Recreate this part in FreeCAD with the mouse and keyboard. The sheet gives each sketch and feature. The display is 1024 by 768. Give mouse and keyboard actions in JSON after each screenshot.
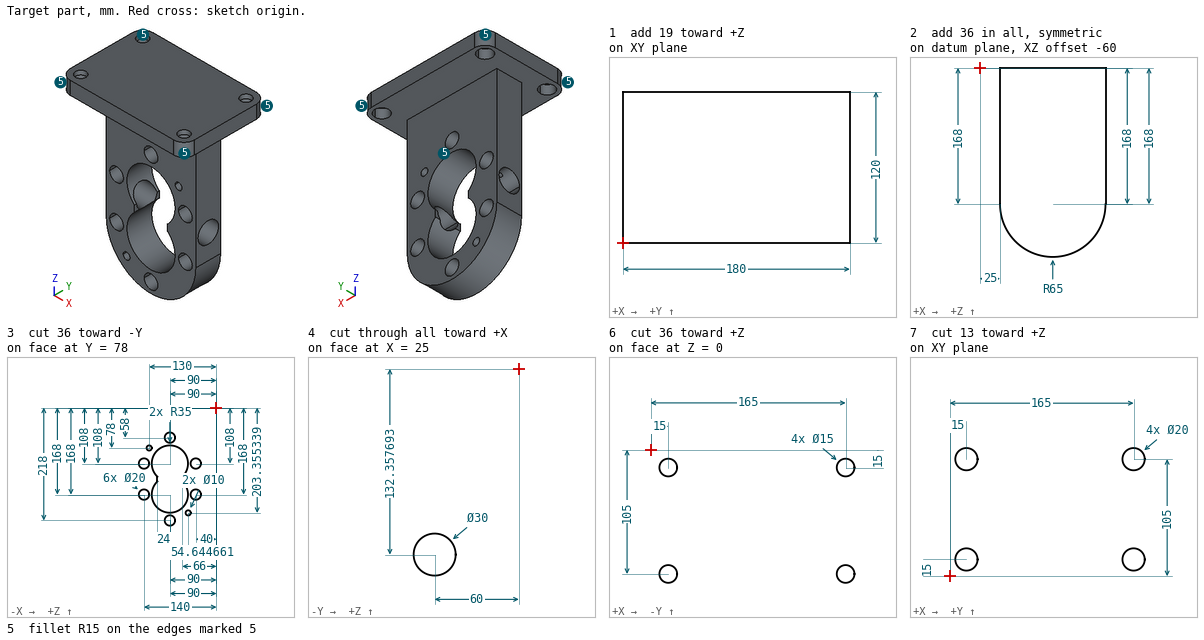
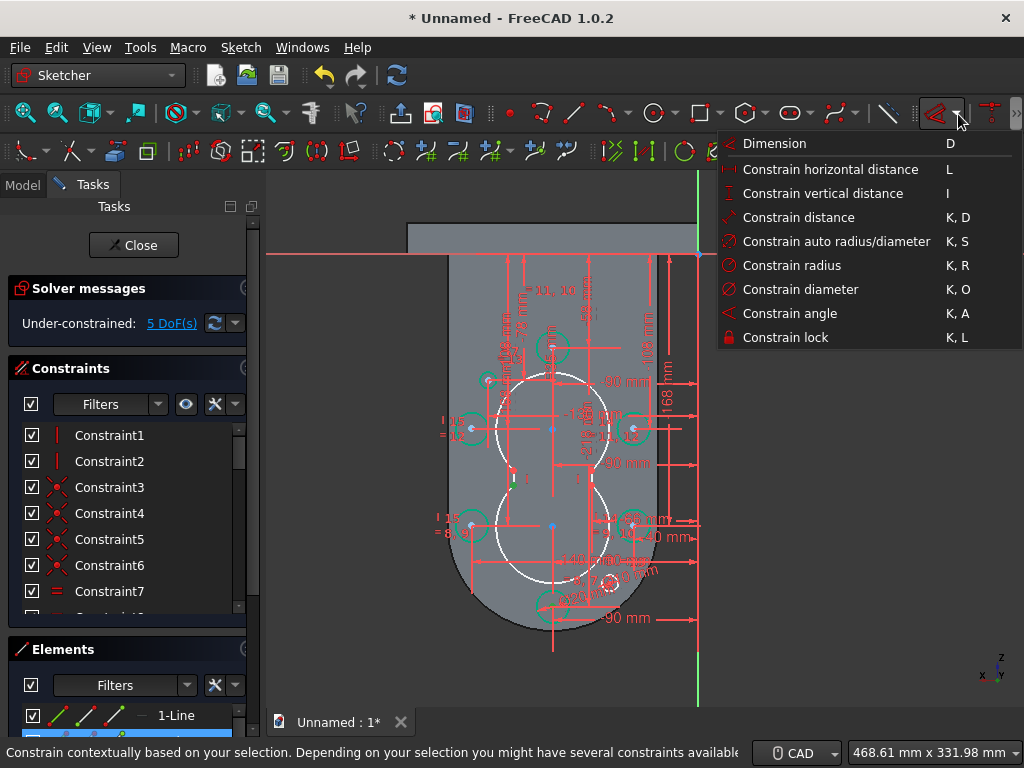
{"action": "left_click", "coordinate": [870, 169]}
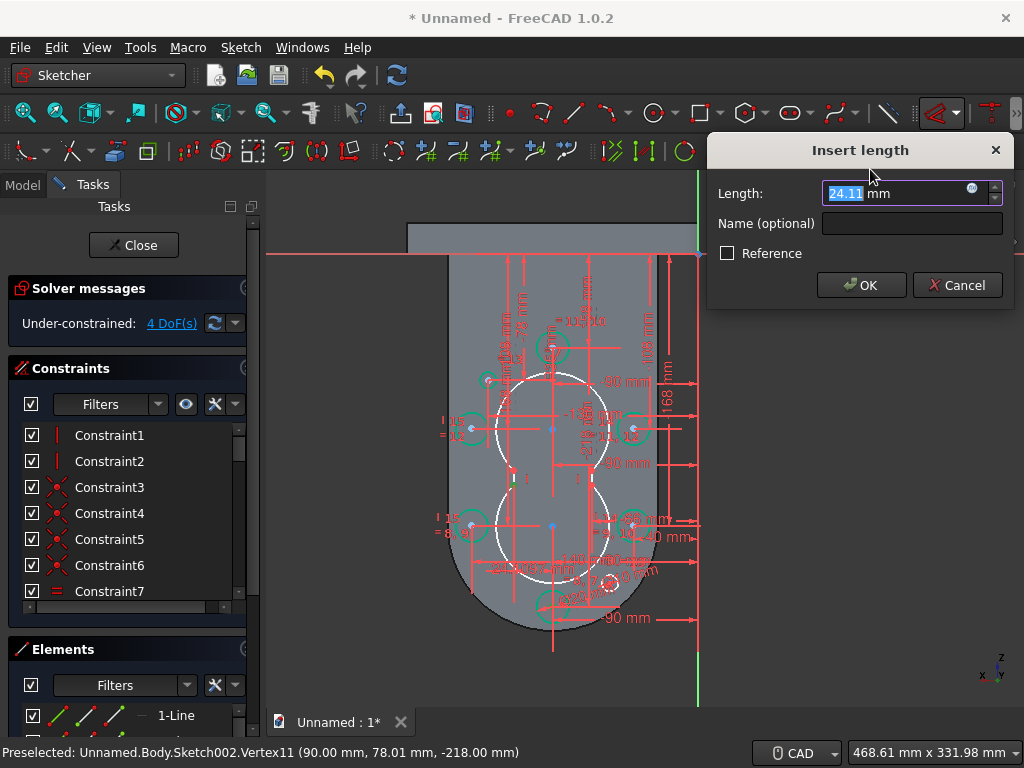
{"action": "type", "text": "24"}
{"action": "key", "text": "Return"}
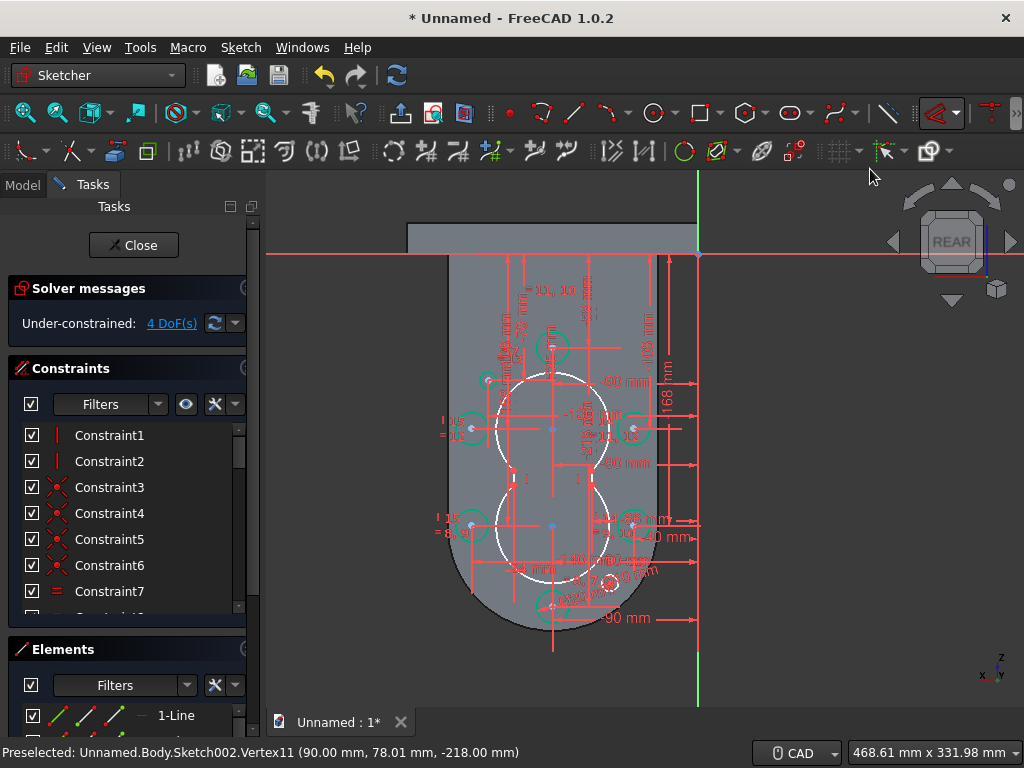
{"action": "left_click", "coordinate": [553, 429]}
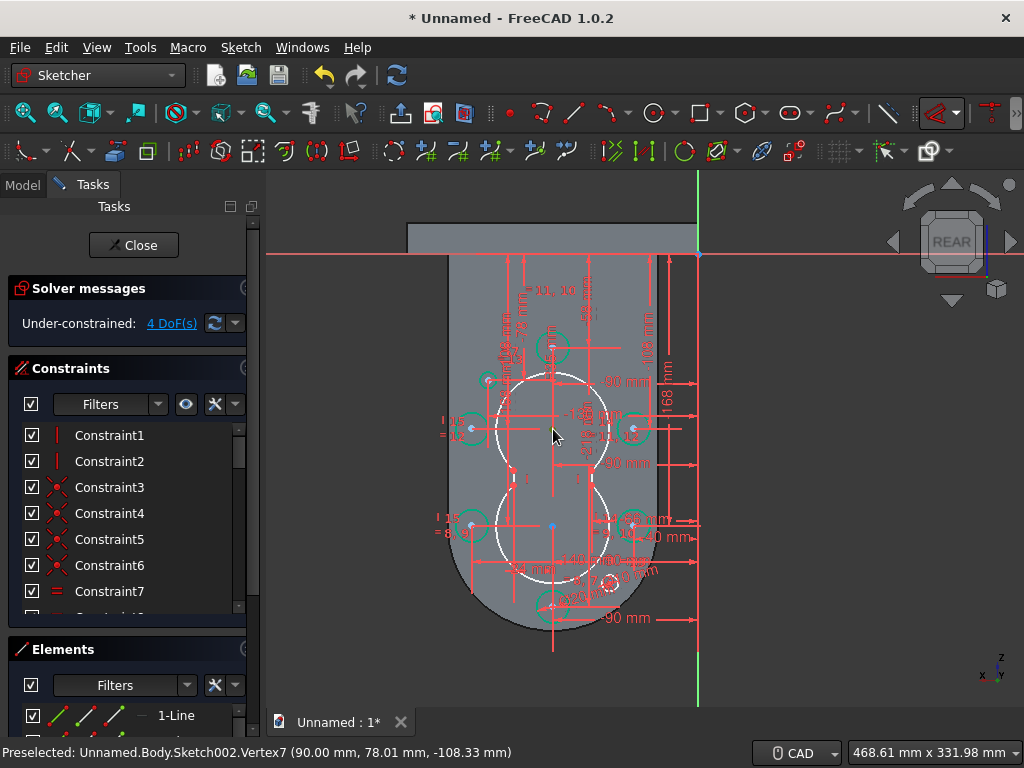
{"action": "left_click", "coordinate": [958, 114]}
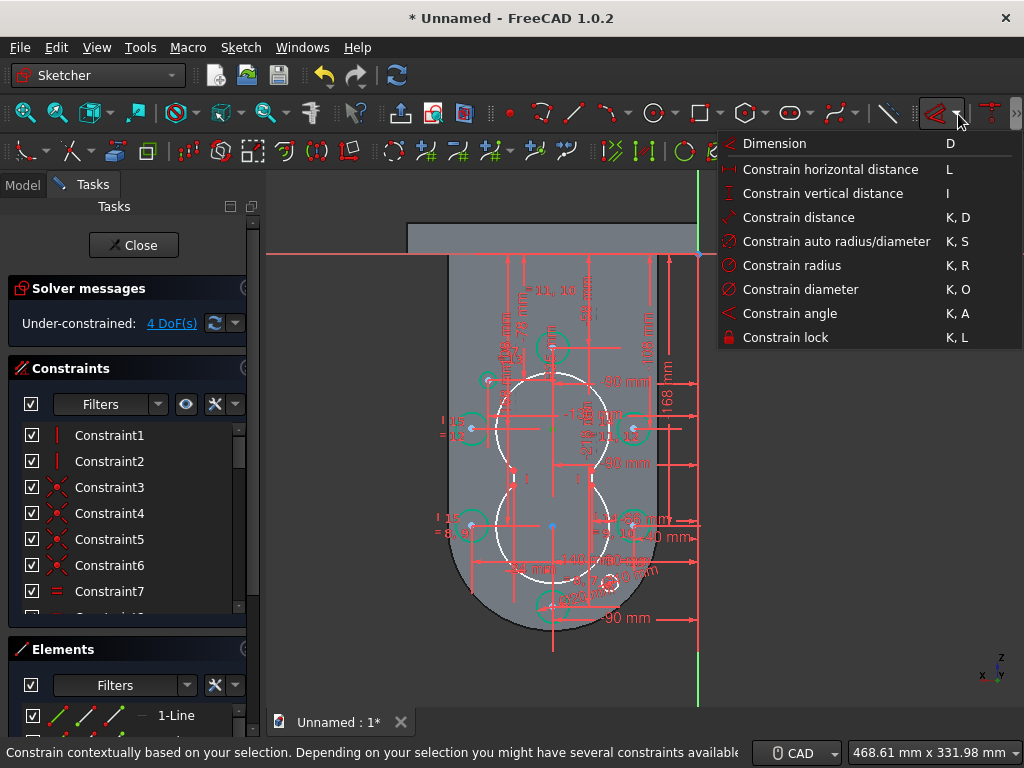
{"action": "left_click", "coordinate": [870, 193]}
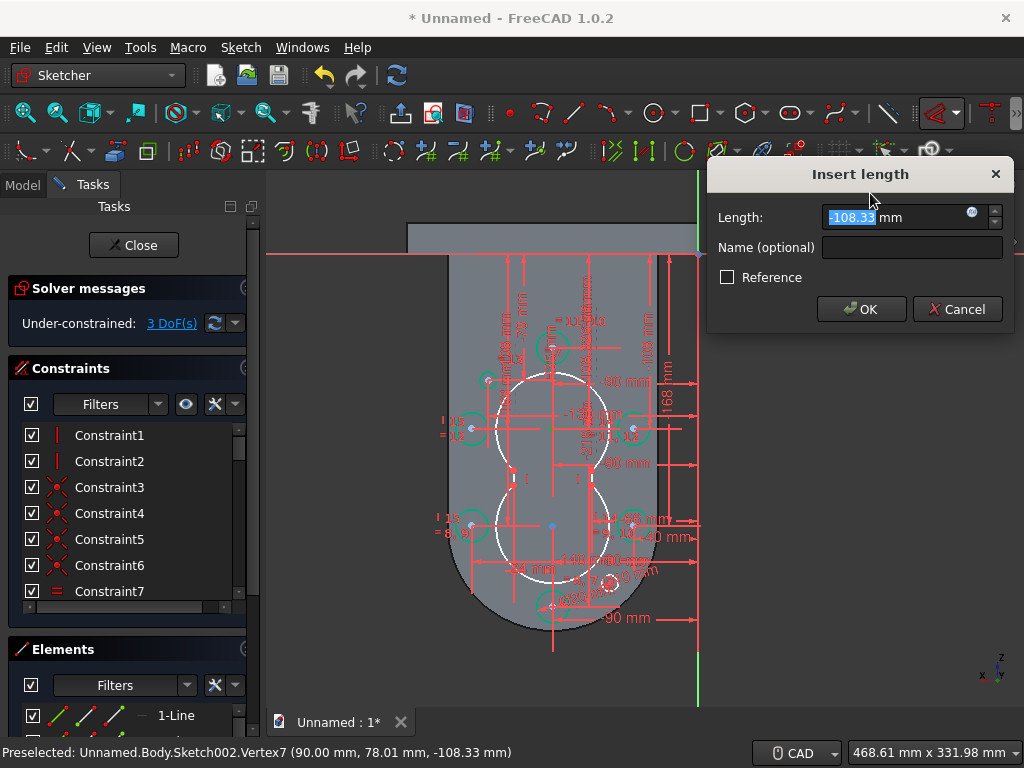
{"action": "type", "text": "-108"}
{"action": "key", "text": "Return"}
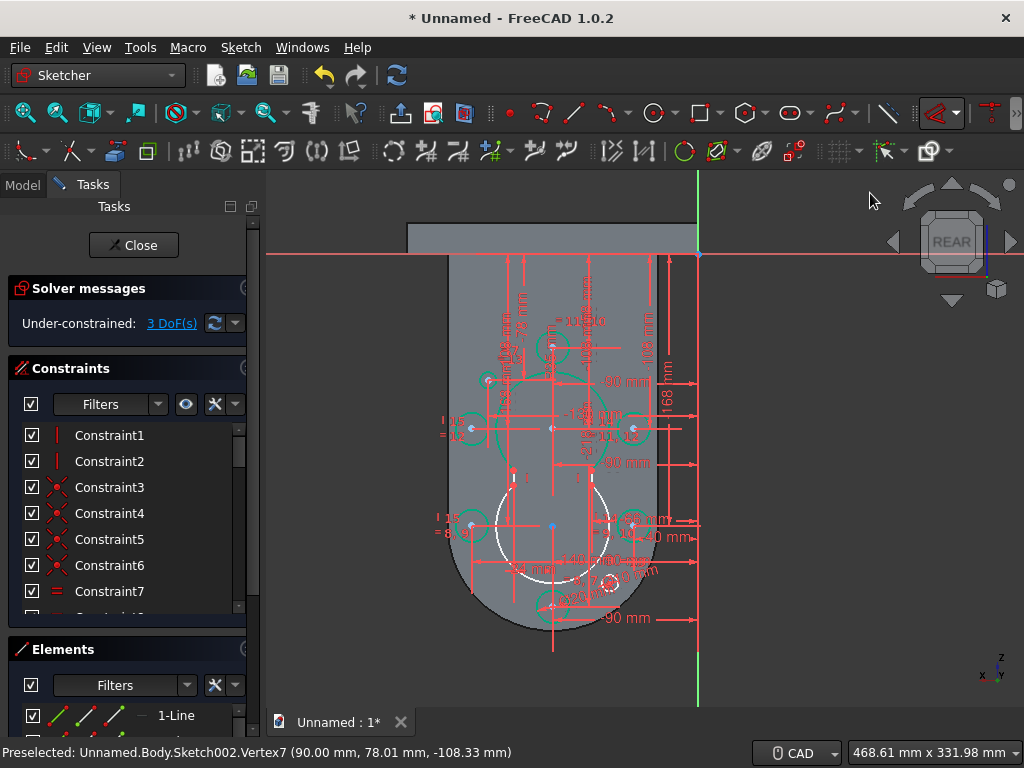
{"action": "left_click", "coordinate": [553, 527]}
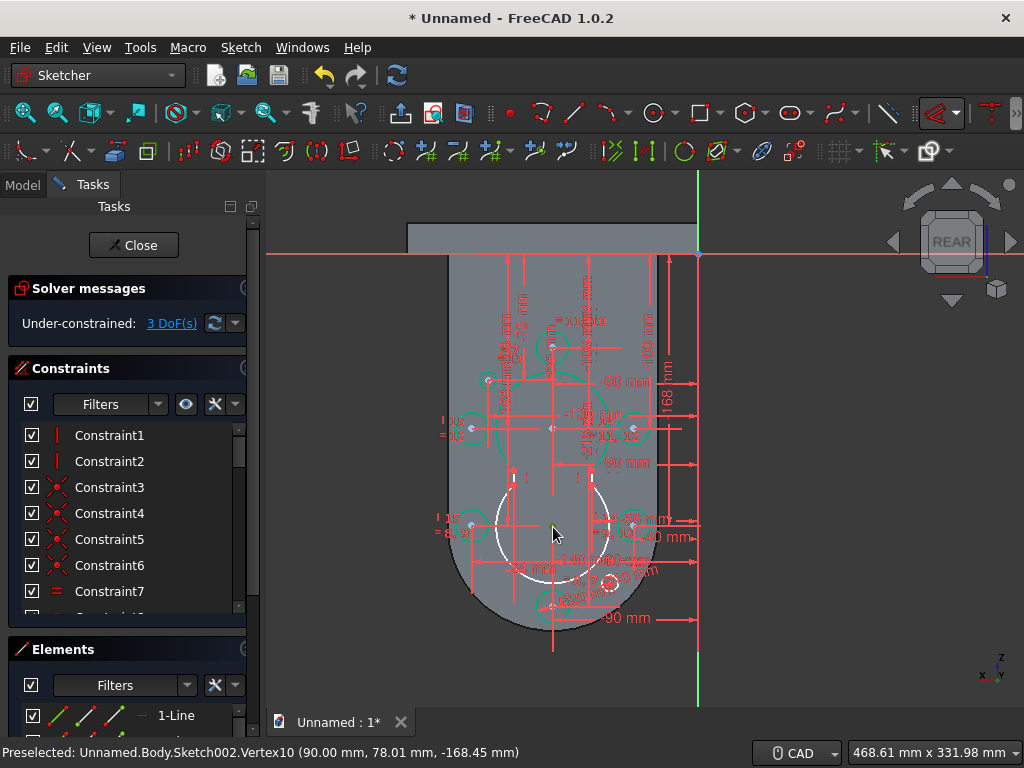
{"action": "key", "text": "i"}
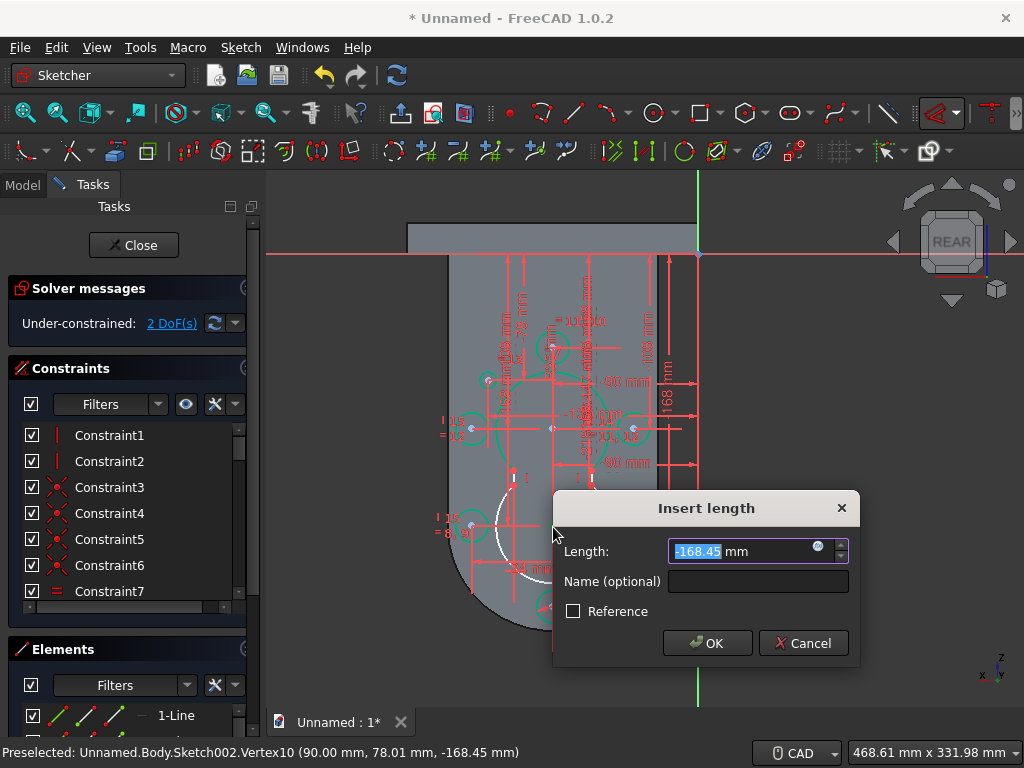
{"action": "type", "text": "-168"}
{"action": "key", "text": "Return"}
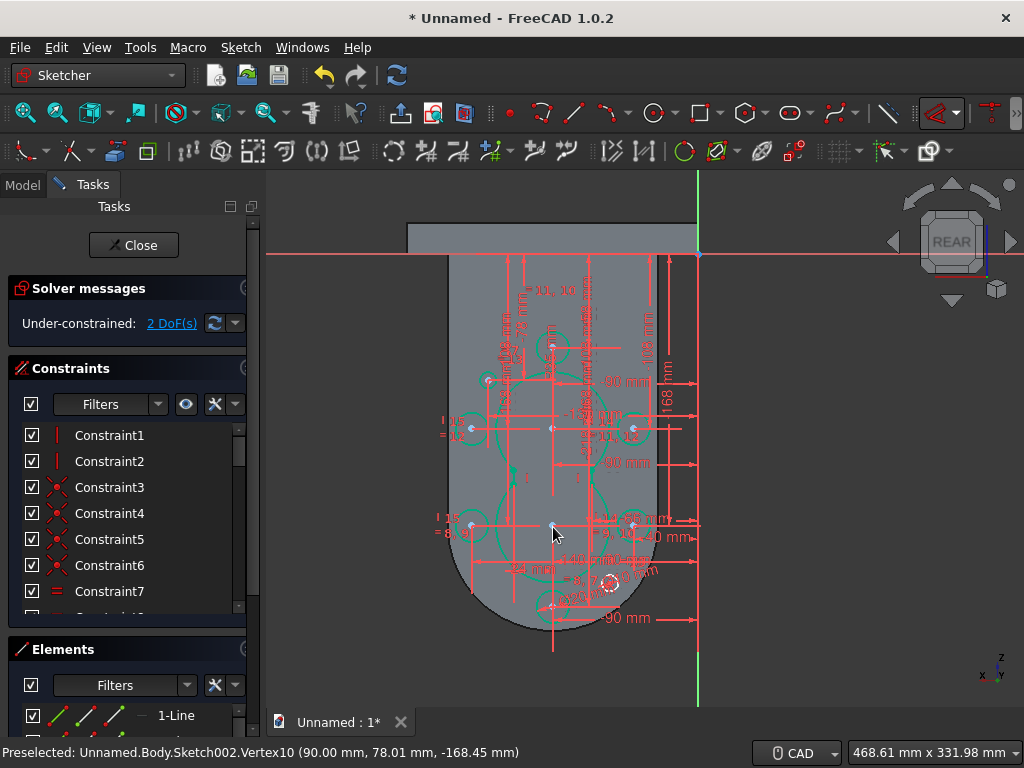
{"action": "left_click", "coordinate": [610, 583]}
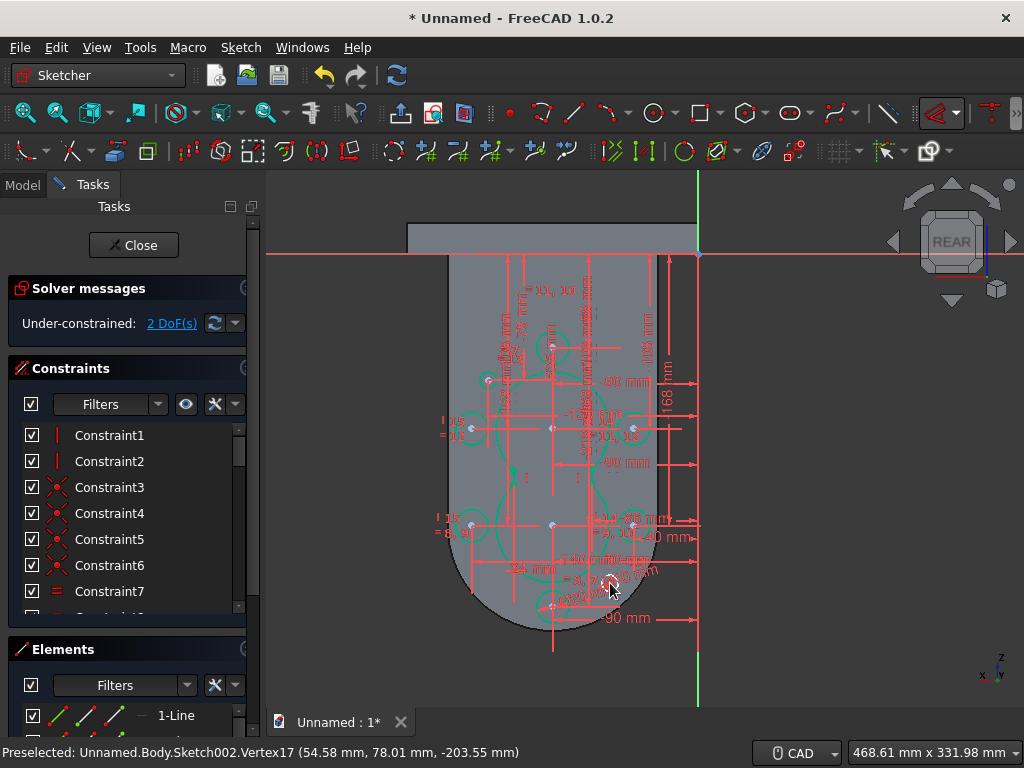
{"action": "left_click", "coordinate": [958, 114]}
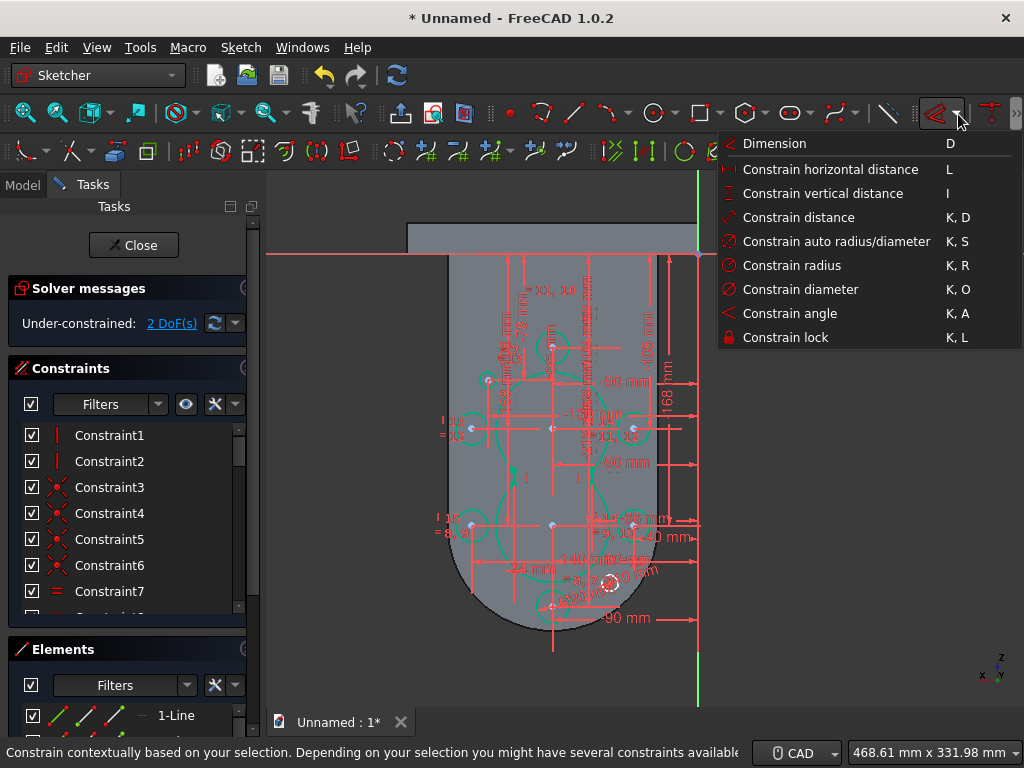
{"action": "left_click", "coordinate": [870, 169]}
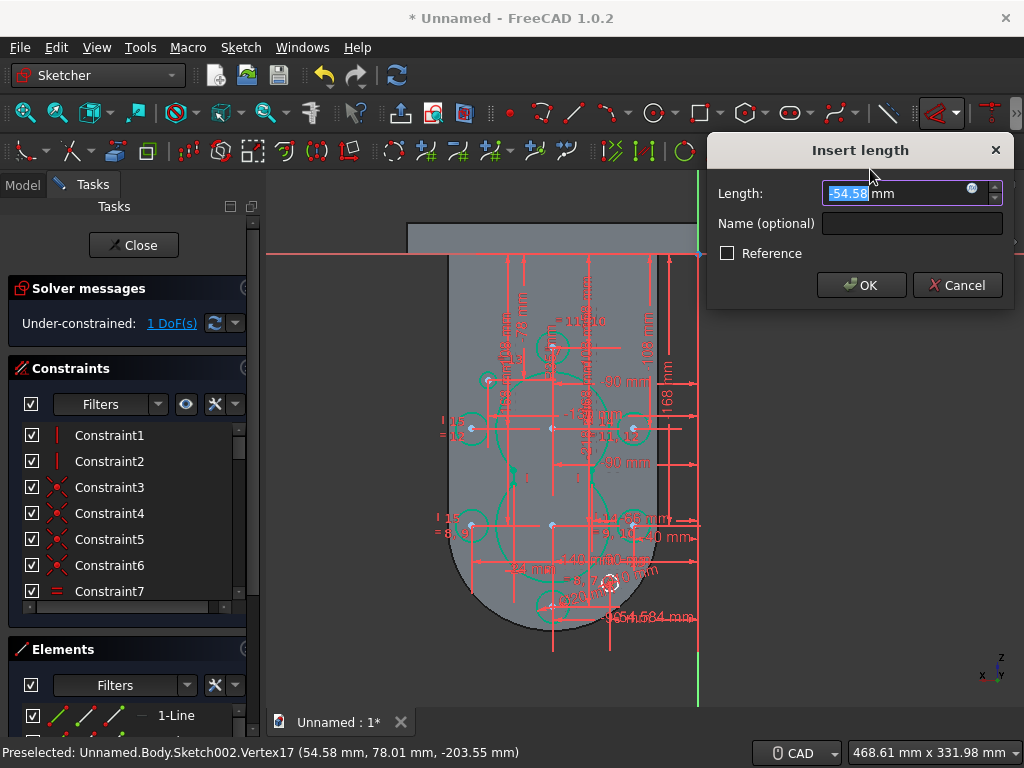
{"action": "type", "text": "-54.644661"}
{"action": "key", "text": "Return"}